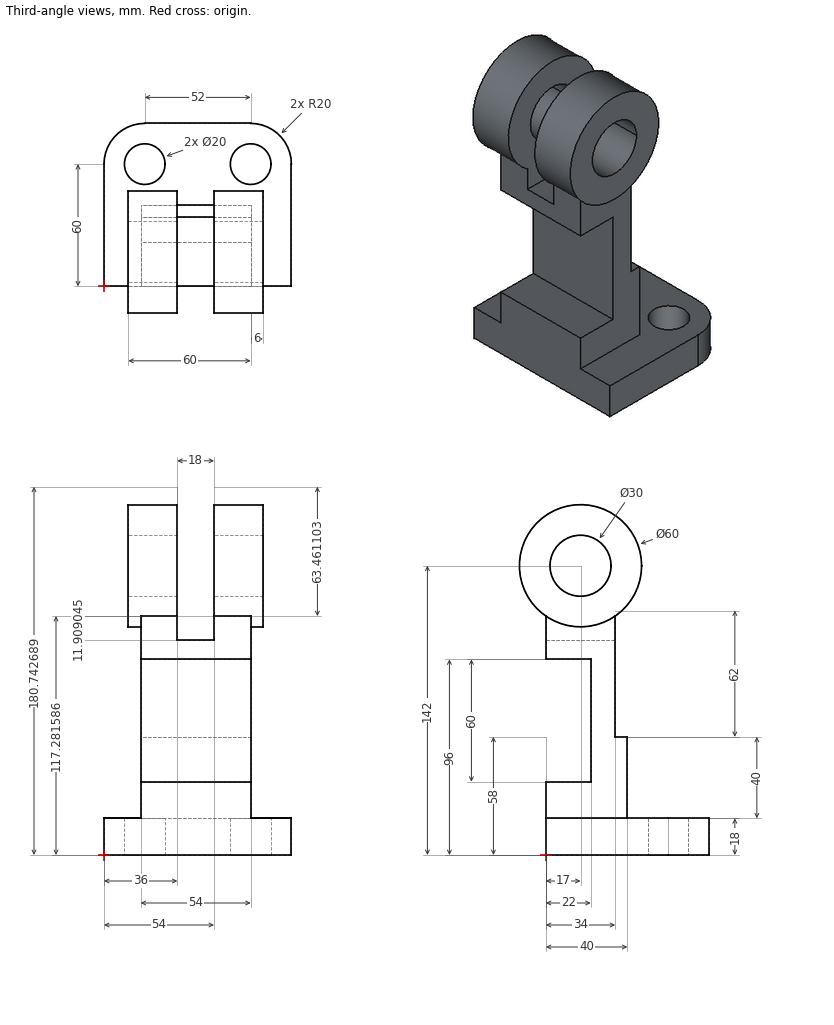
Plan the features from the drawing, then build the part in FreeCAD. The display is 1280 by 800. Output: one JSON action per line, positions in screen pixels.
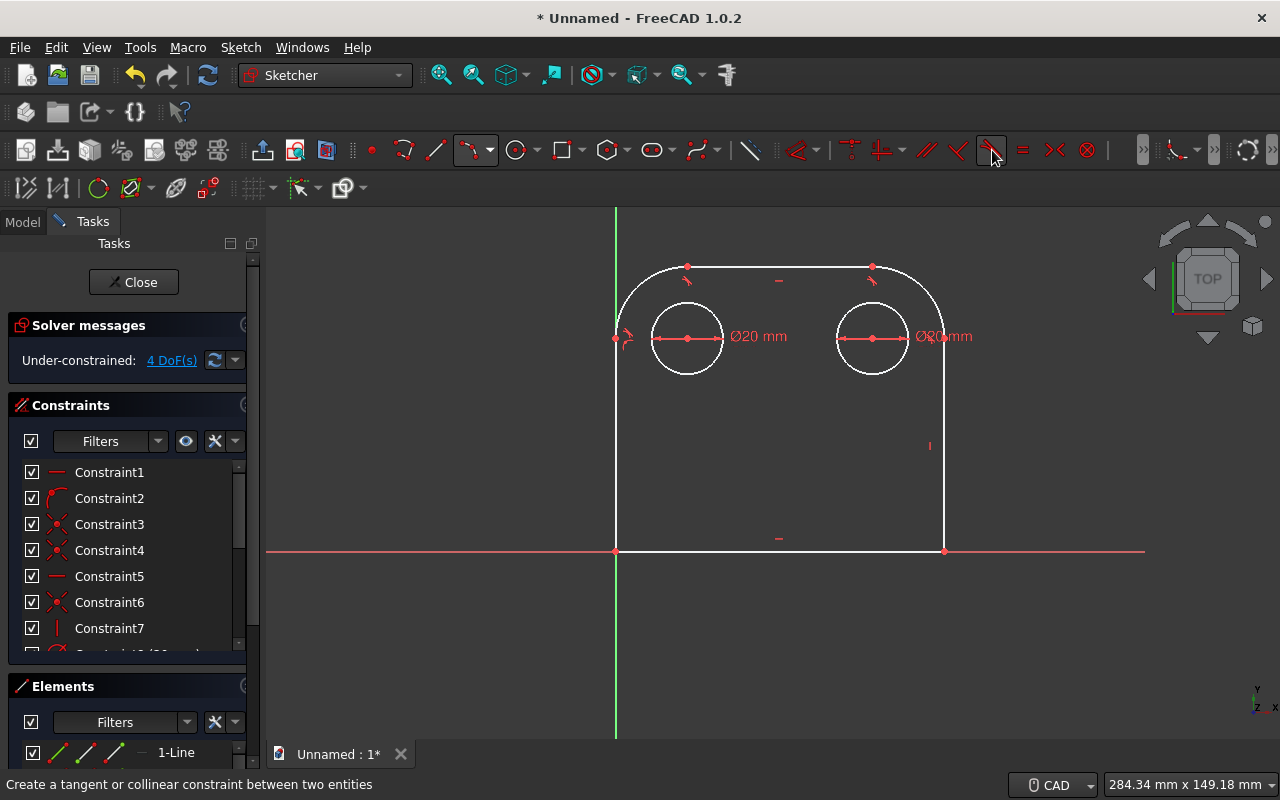
{"action": "left_click", "coordinate": [655, 275]}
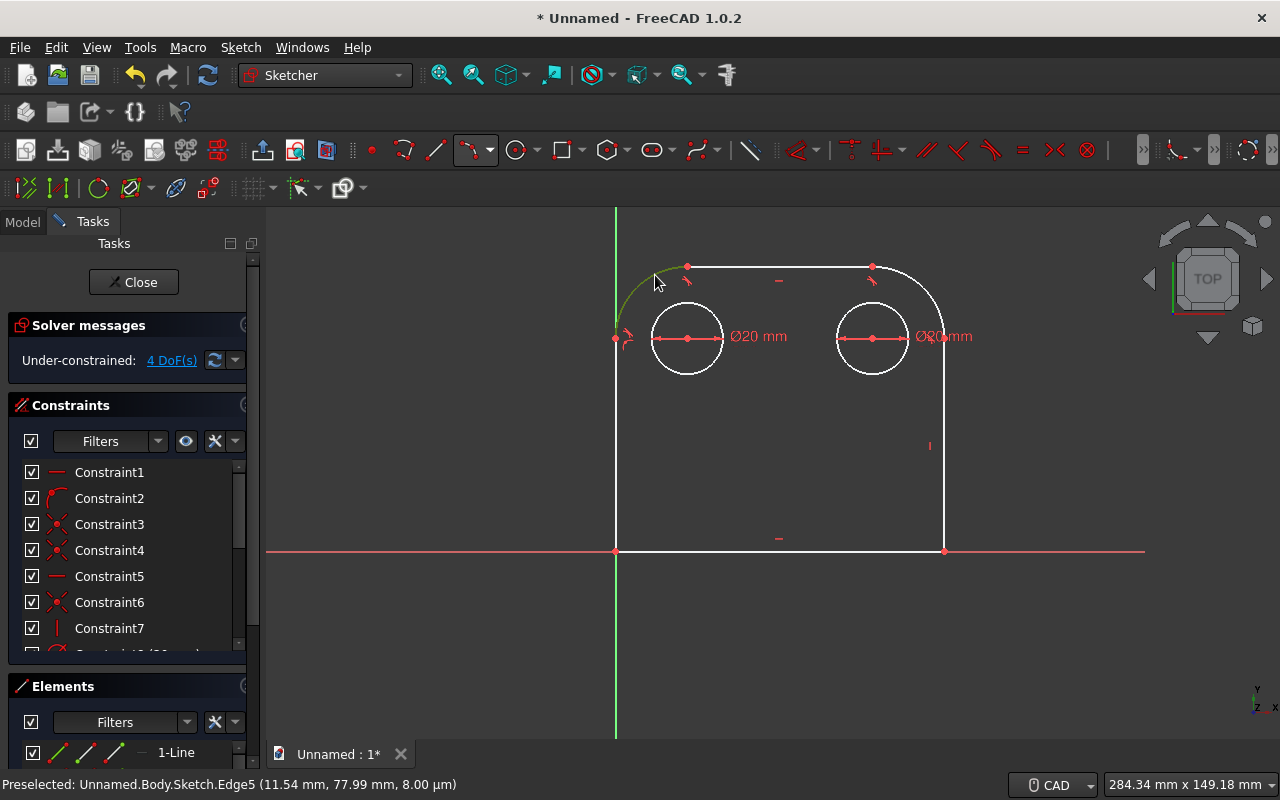
{"action": "left_click", "coordinate": [936, 306]}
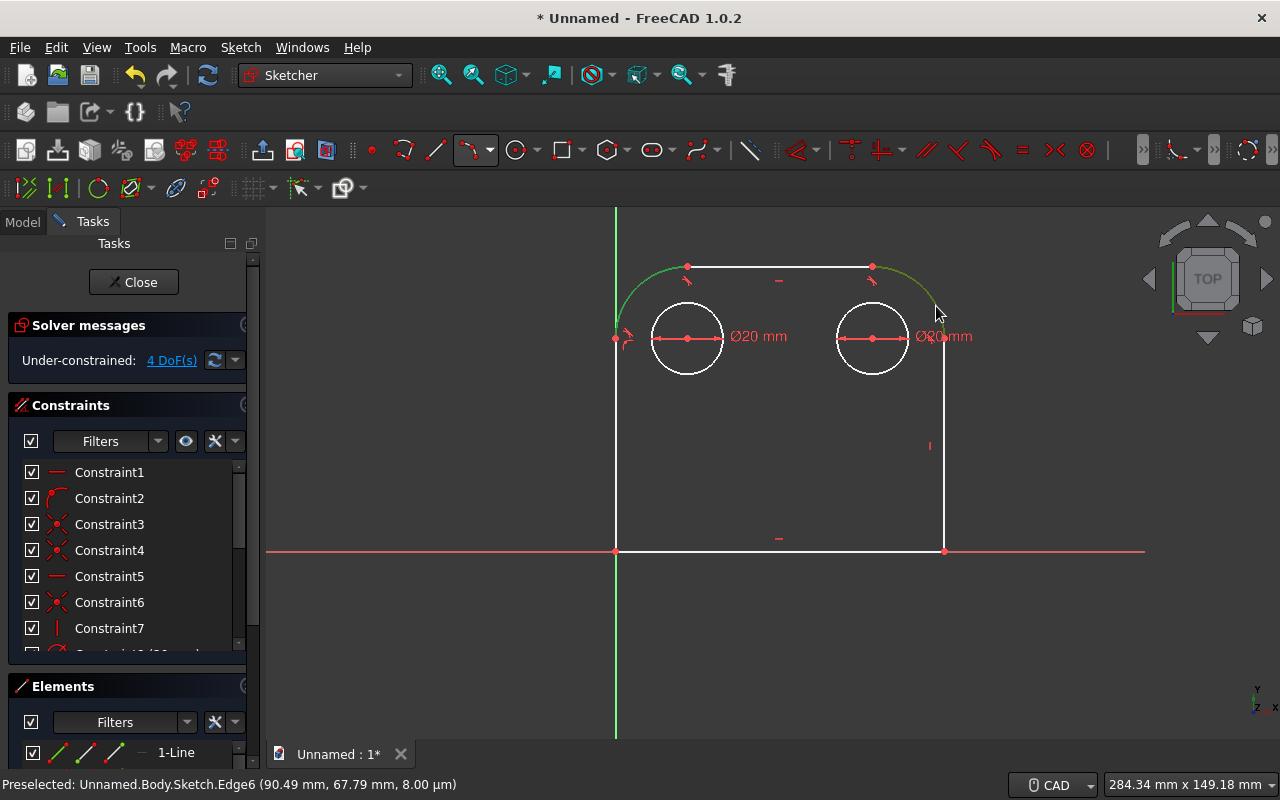
{"action": "left_click", "coordinate": [1024, 150]}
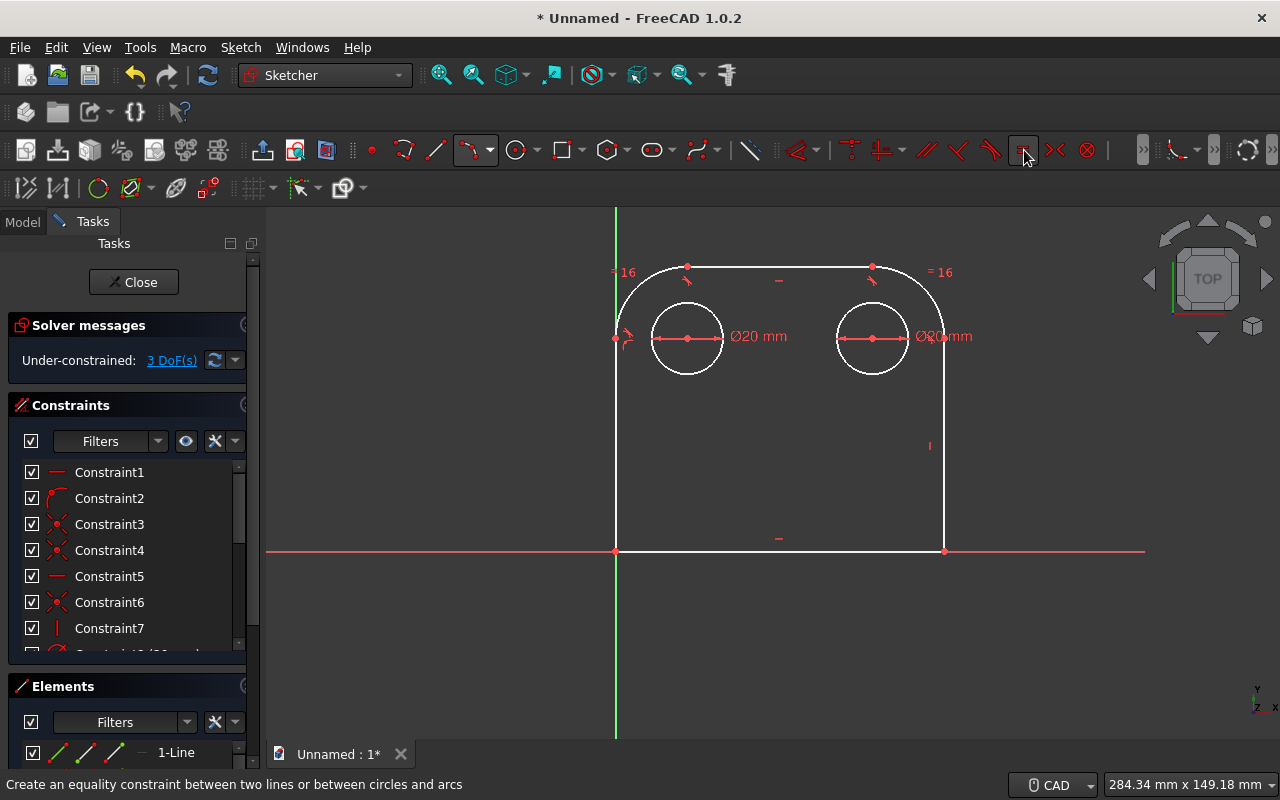
{"action": "left_click", "coordinate": [655, 275]}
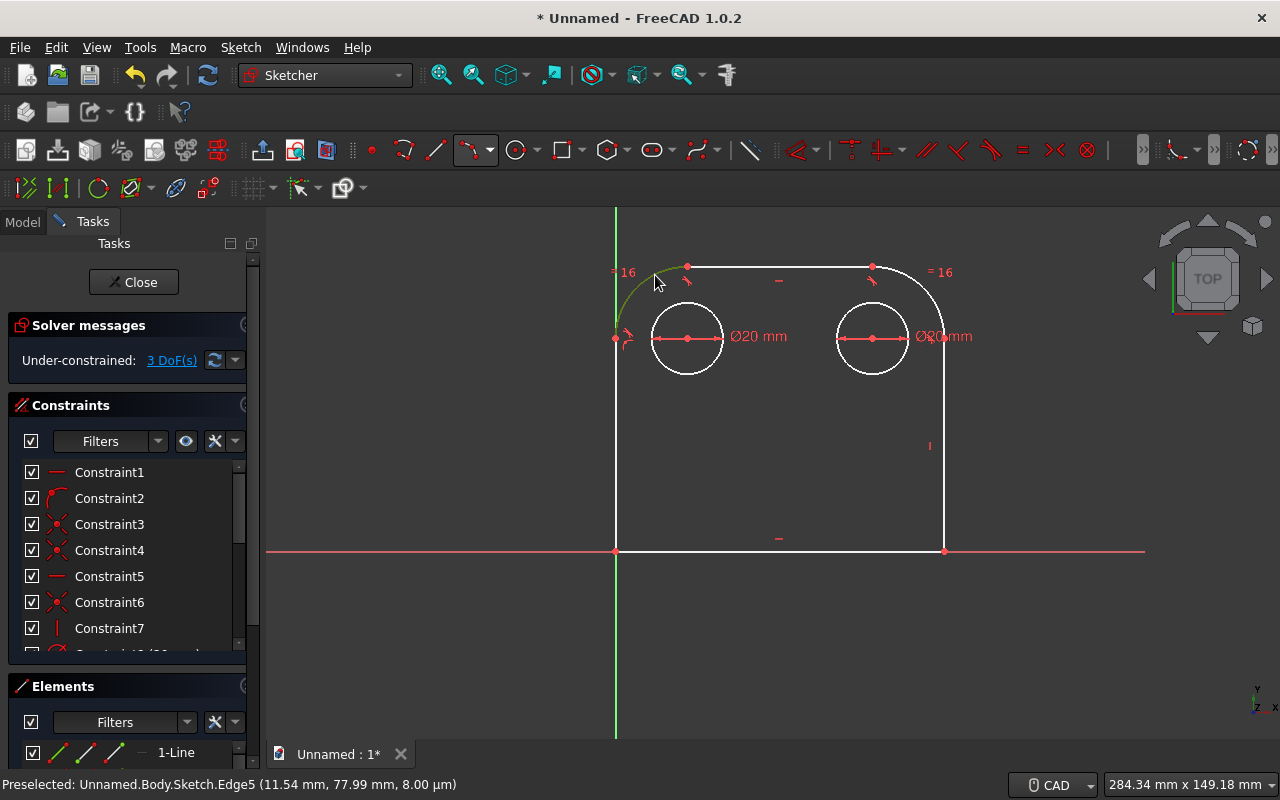
{"action": "left_click", "coordinate": [818, 150]}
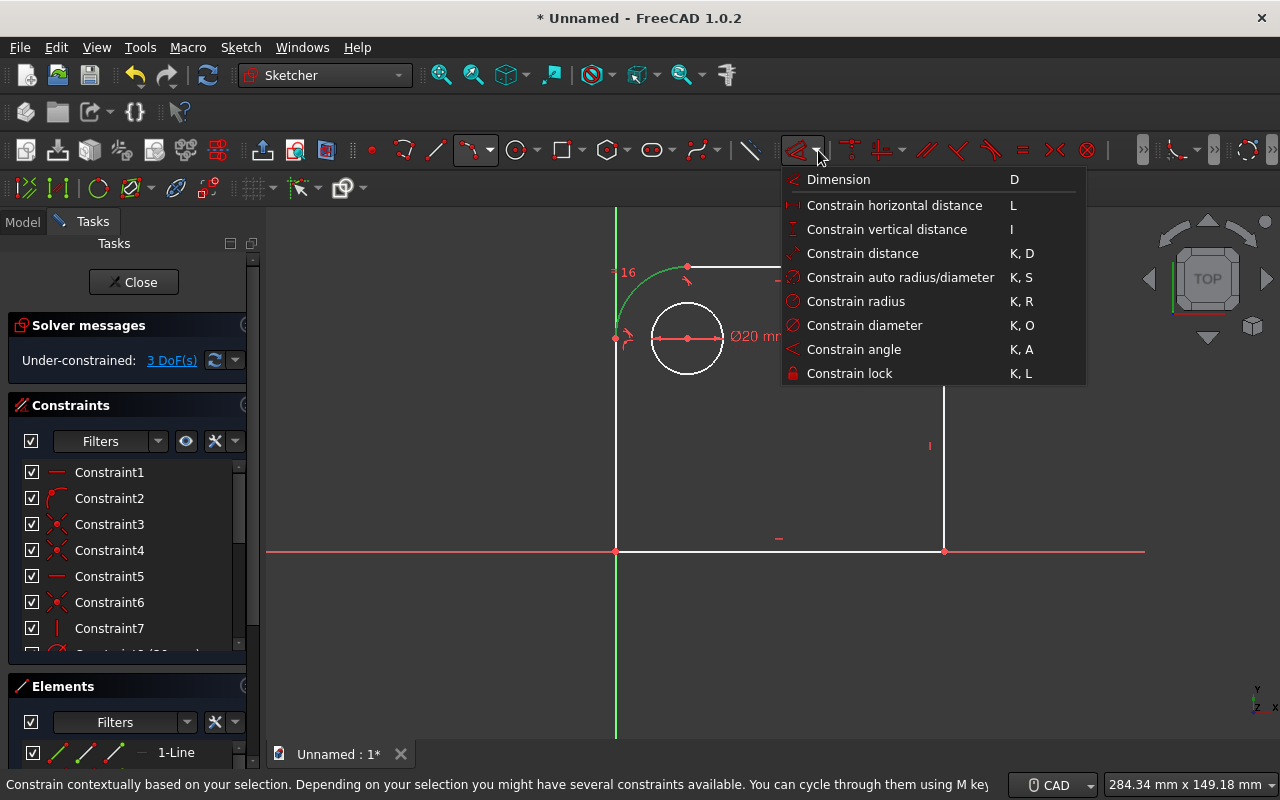
{"action": "left_click", "coordinate": [934, 301]}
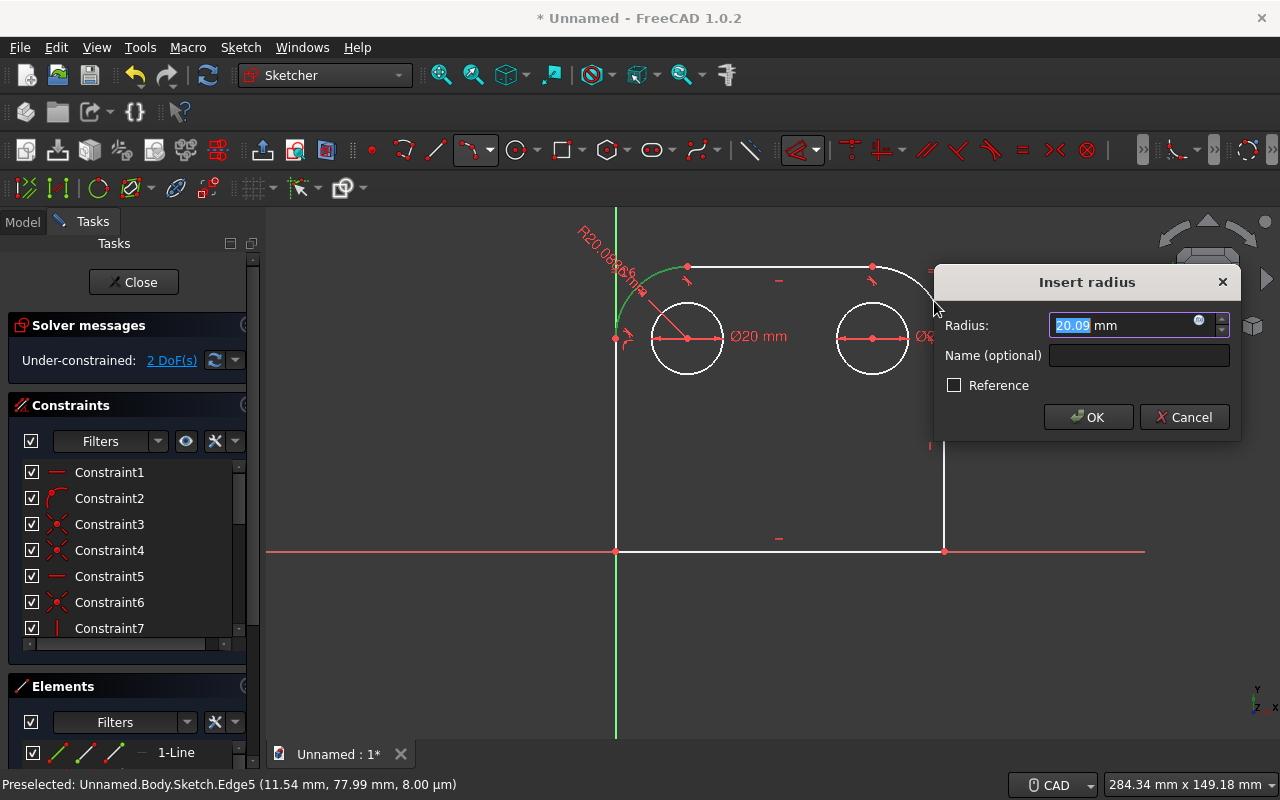
{"action": "type", "text": "20"}
{"action": "key", "text": "Return"}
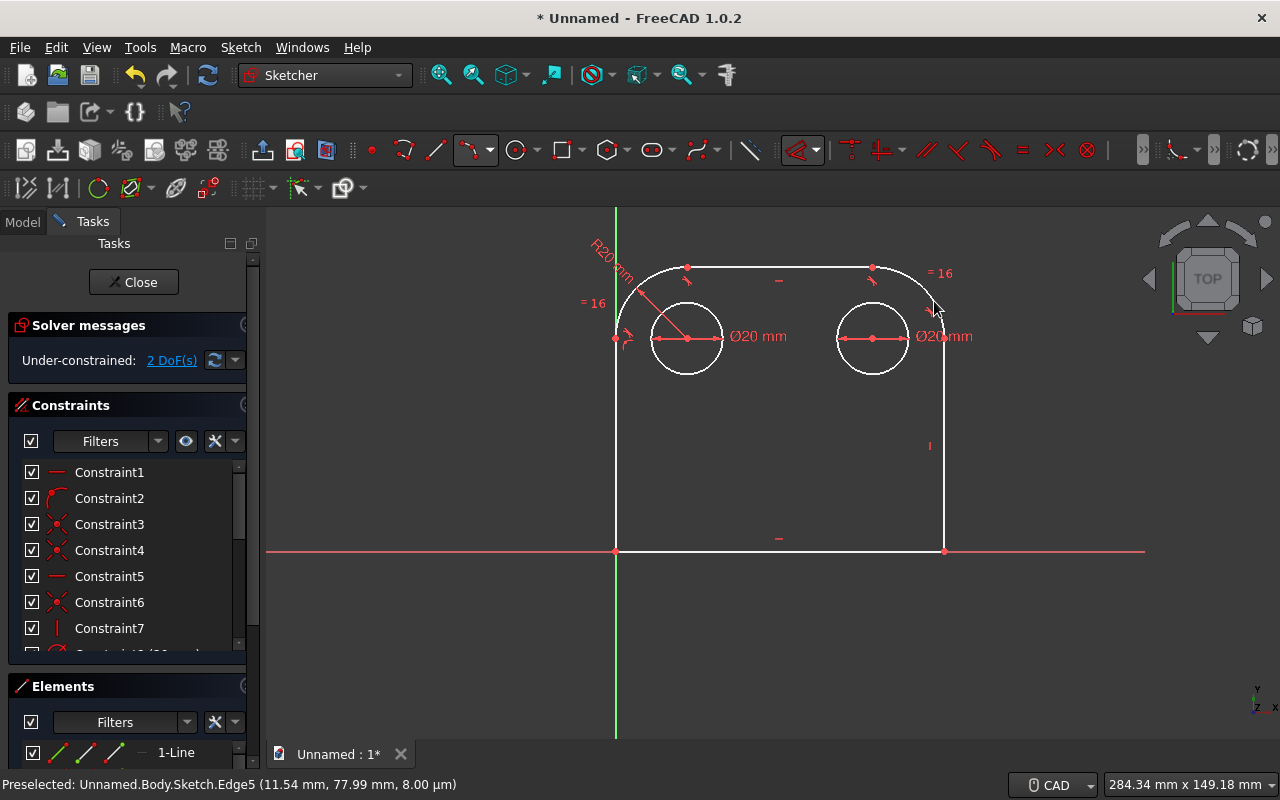
{"action": "left_click", "coordinate": [817, 267]}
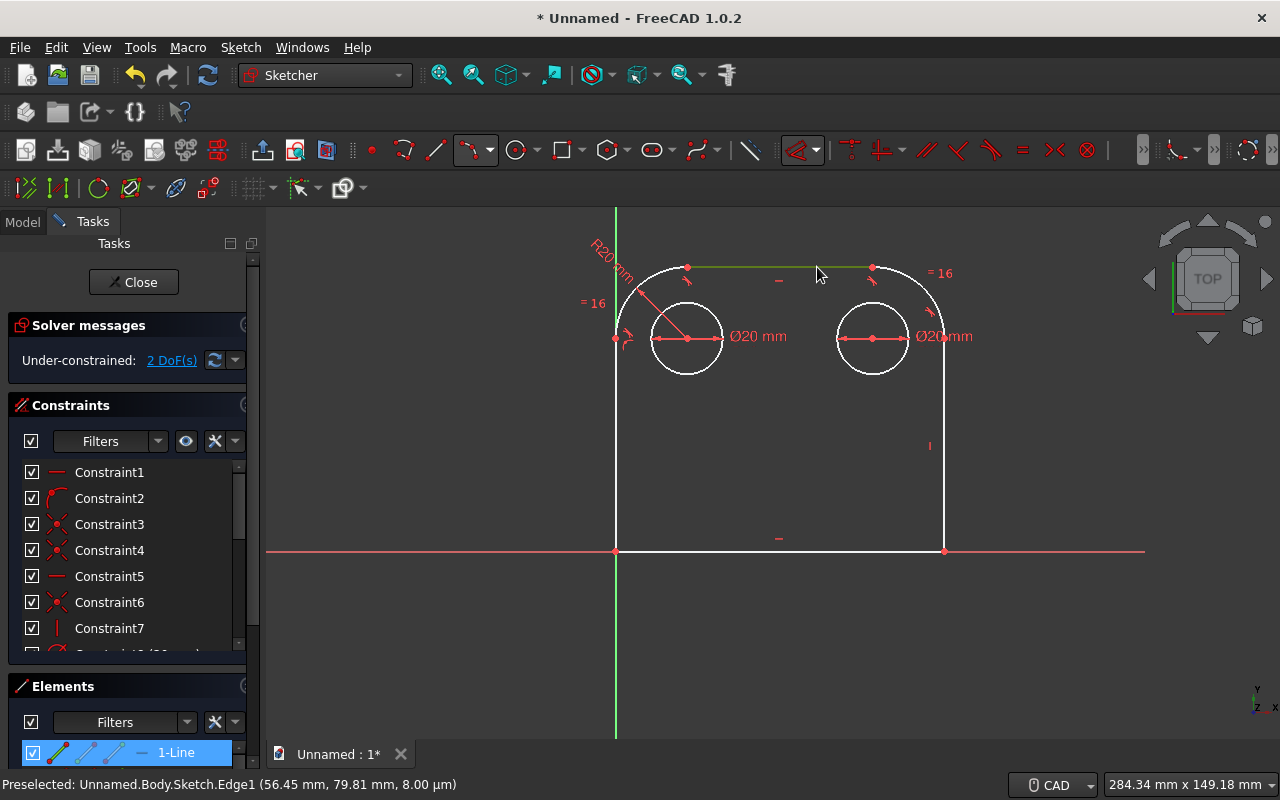
{"action": "left_click", "coordinate": [818, 150]}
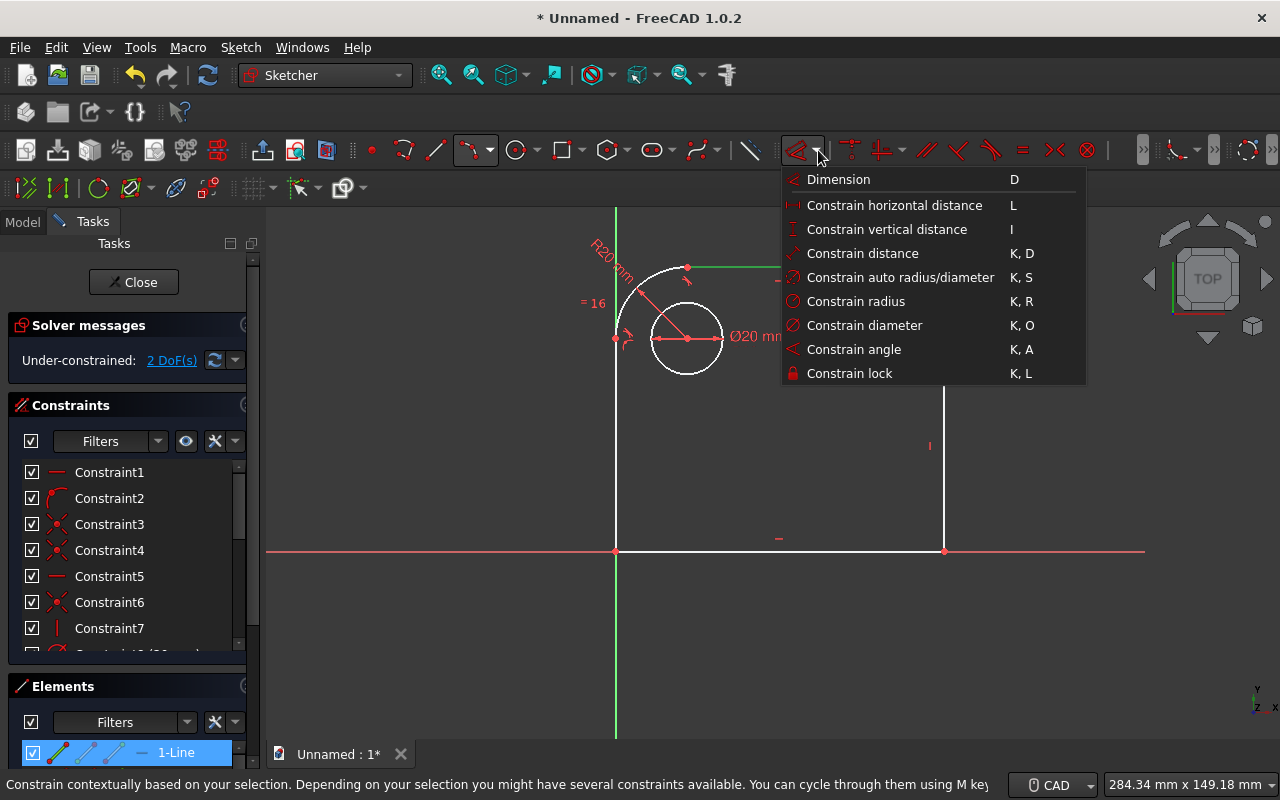
{"action": "left_click", "coordinate": [934, 205]}